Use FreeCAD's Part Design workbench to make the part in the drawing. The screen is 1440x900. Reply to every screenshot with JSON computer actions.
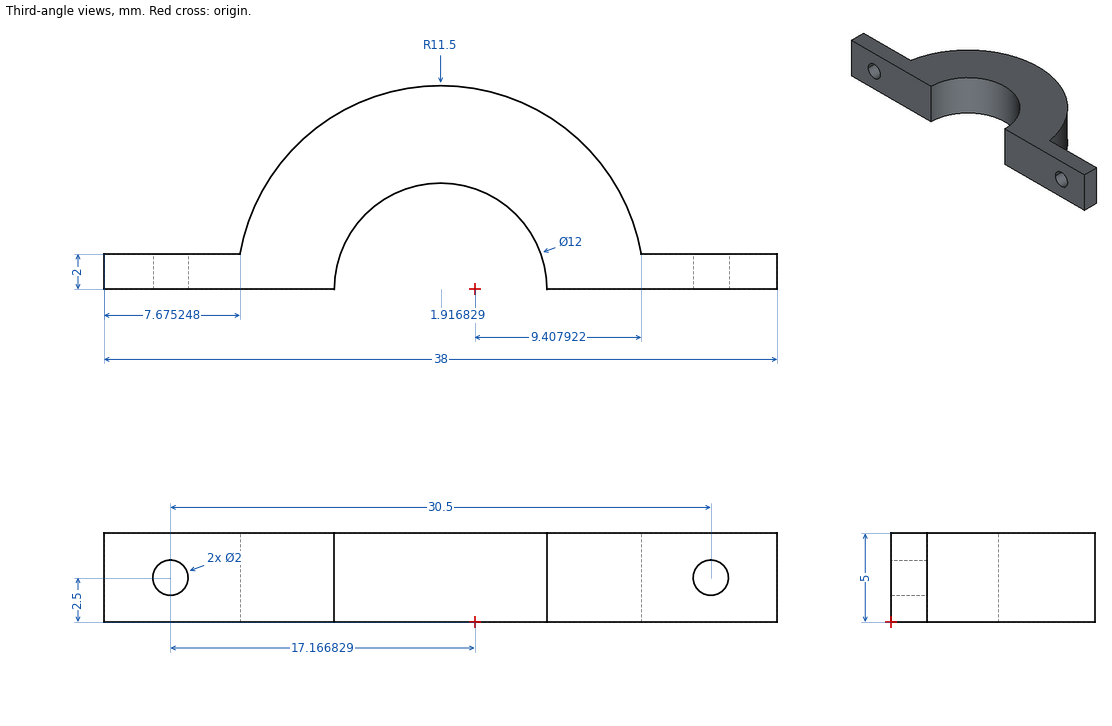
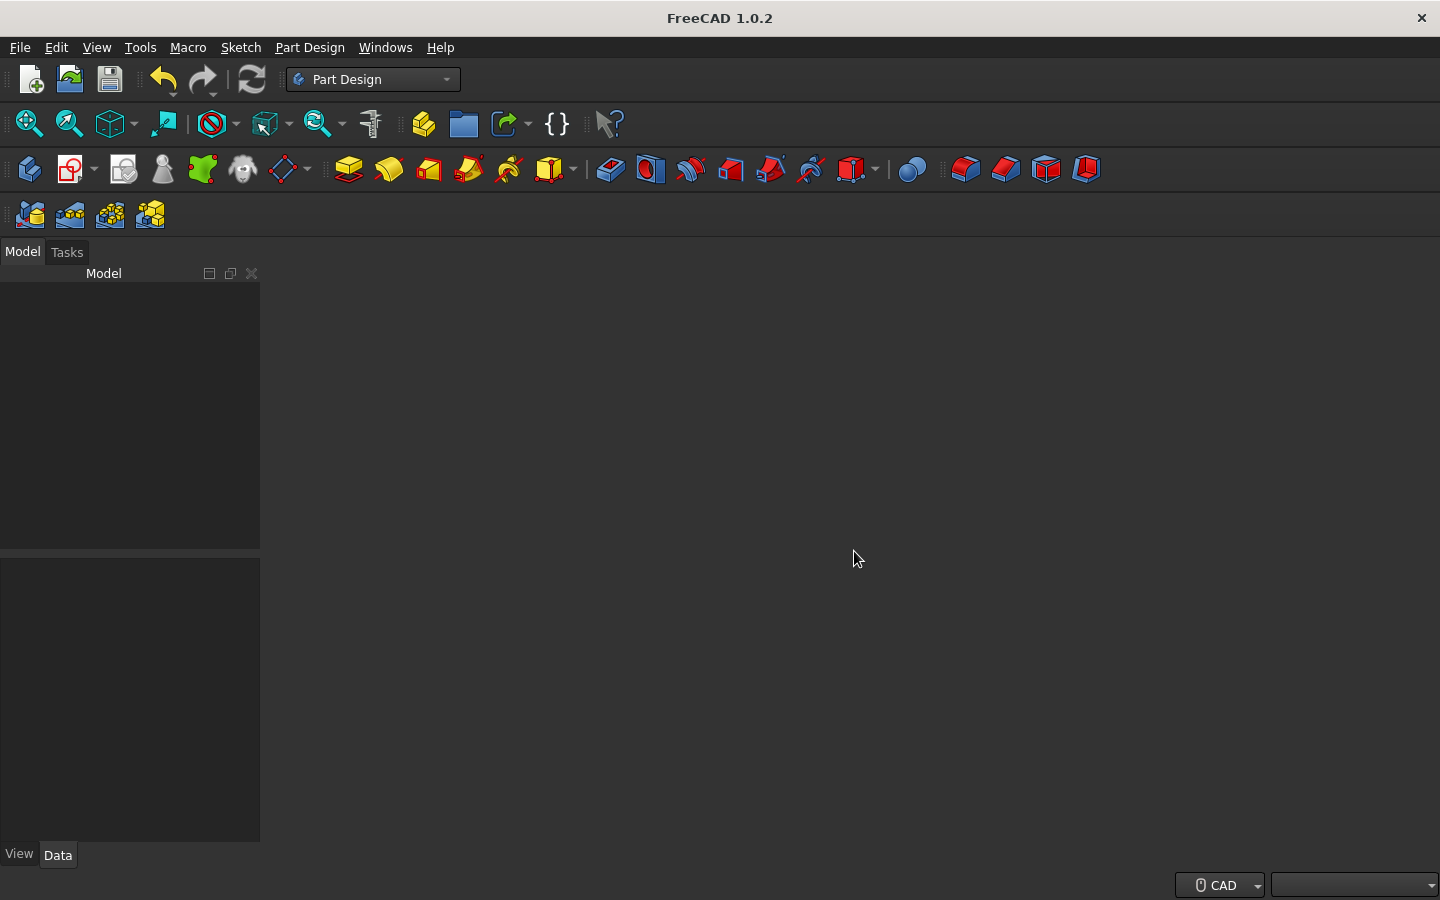
{"action": "left_click", "coordinate": [30, 80]}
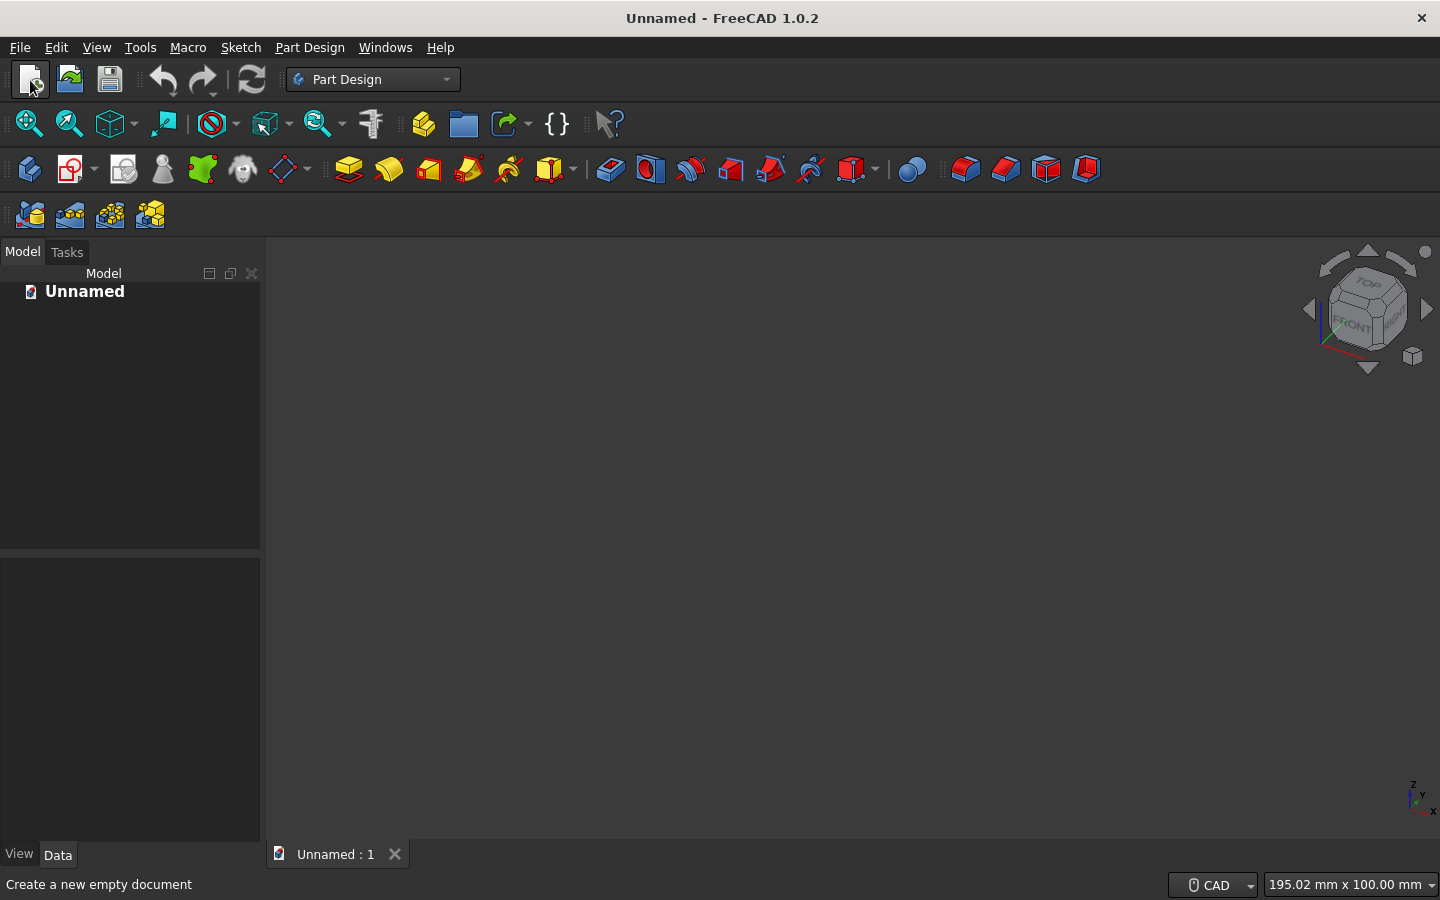
{"action": "left_click", "coordinate": [70, 170]}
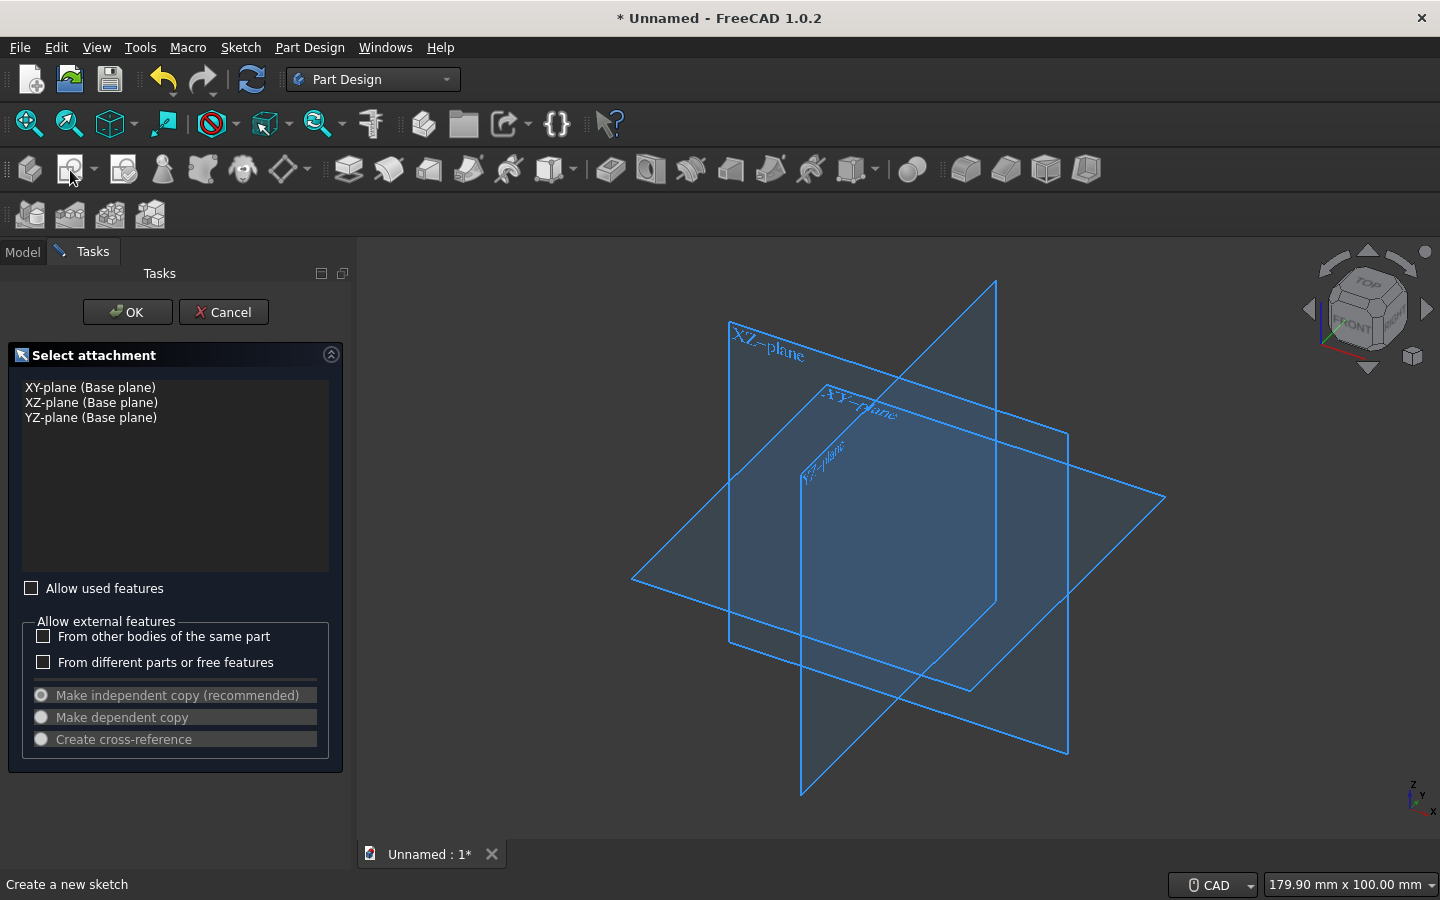
{"action": "left_click", "coordinate": [82, 388]}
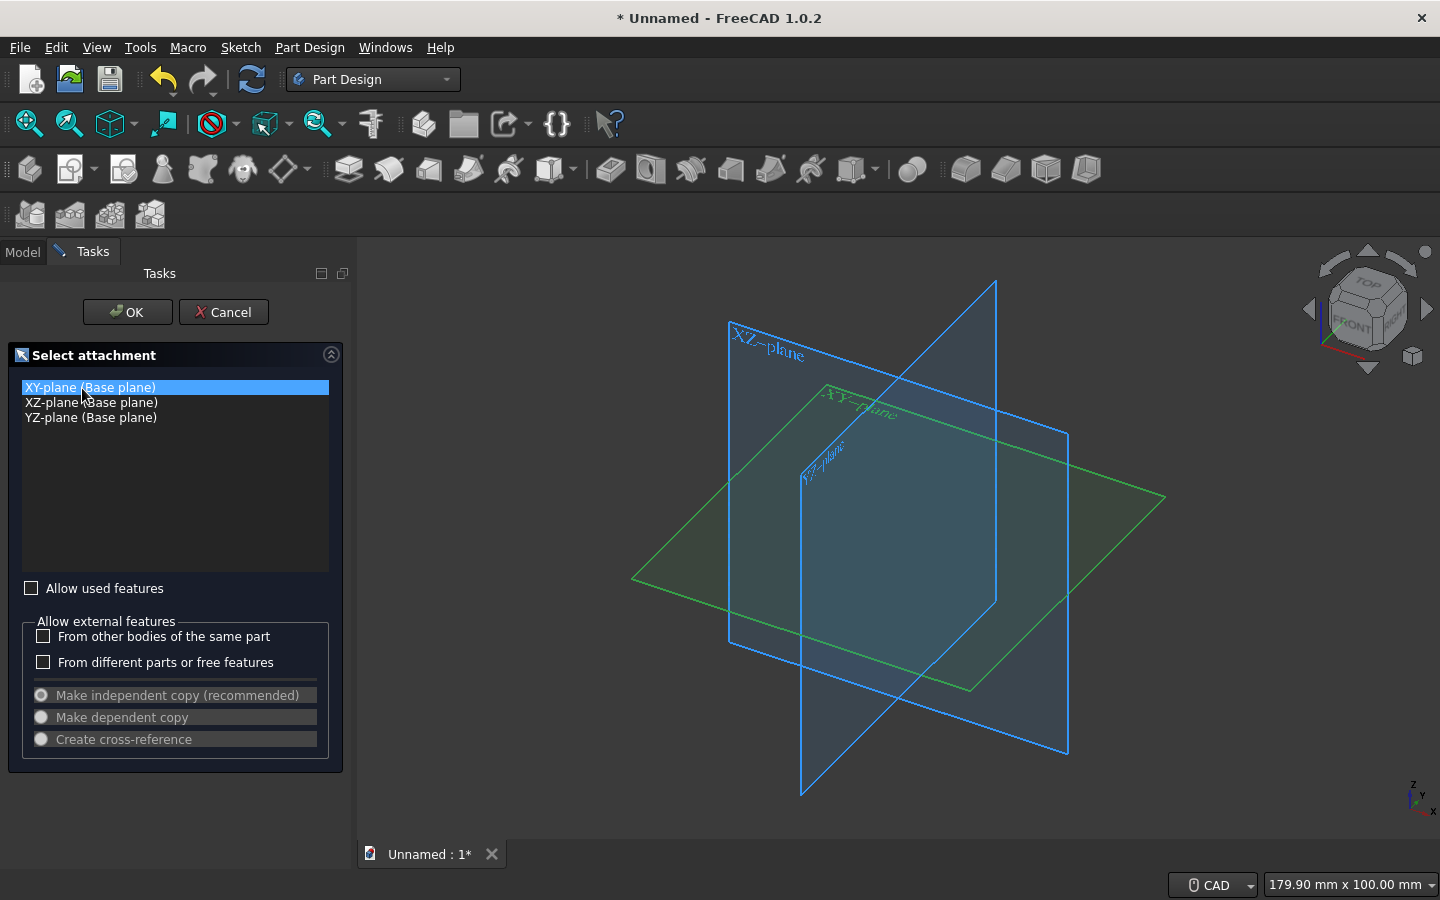
{"action": "left_click", "coordinate": [128, 312]}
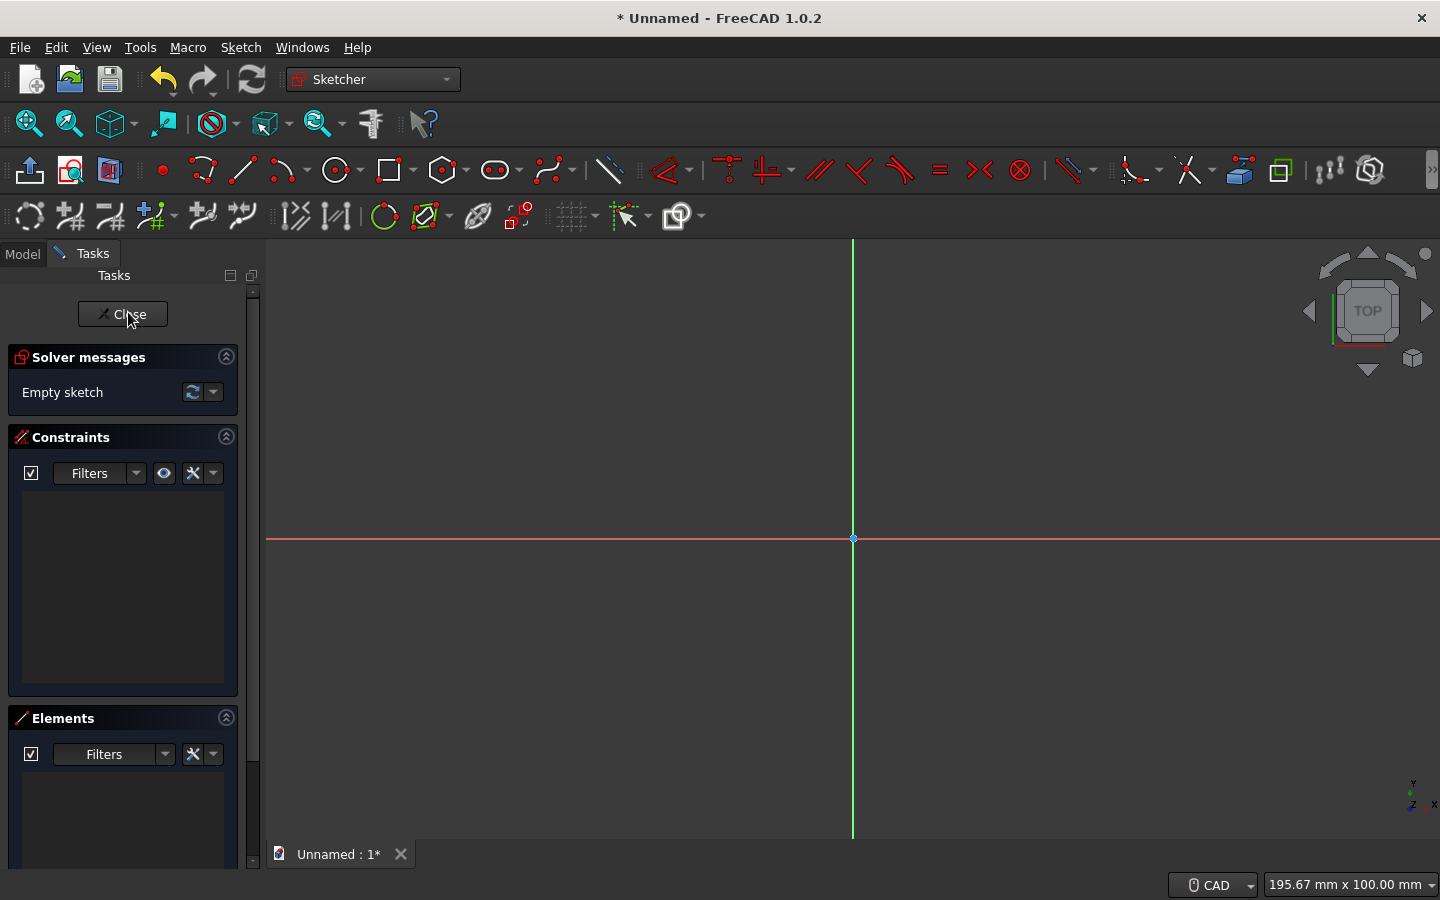
{"action": "scroll", "coordinate": [866, 490], "scroll_direction": "up", "scroll_amount": 6}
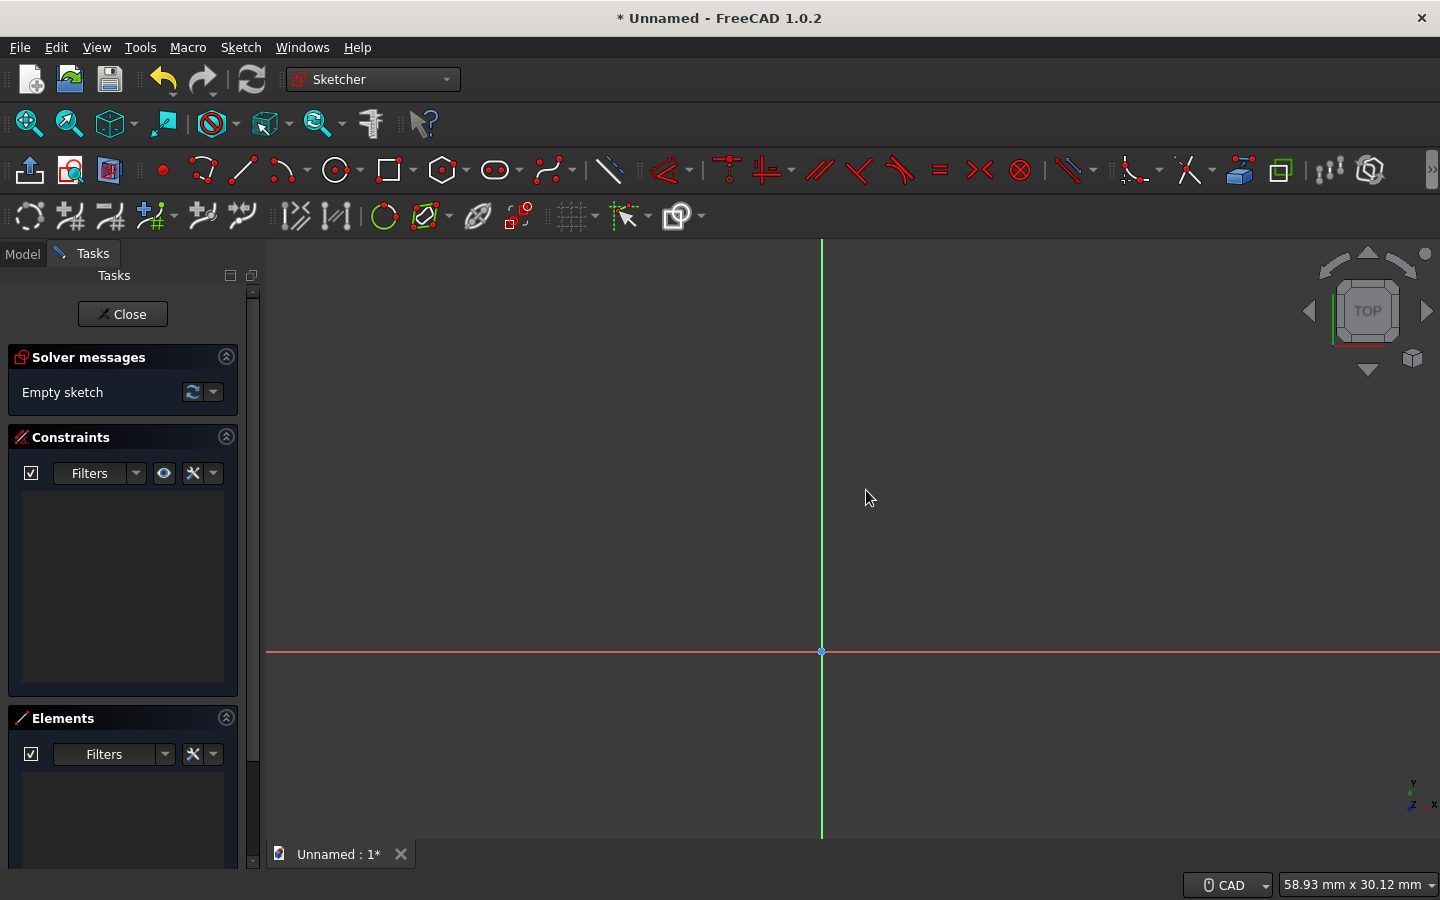
{"action": "key", "text": "g m"}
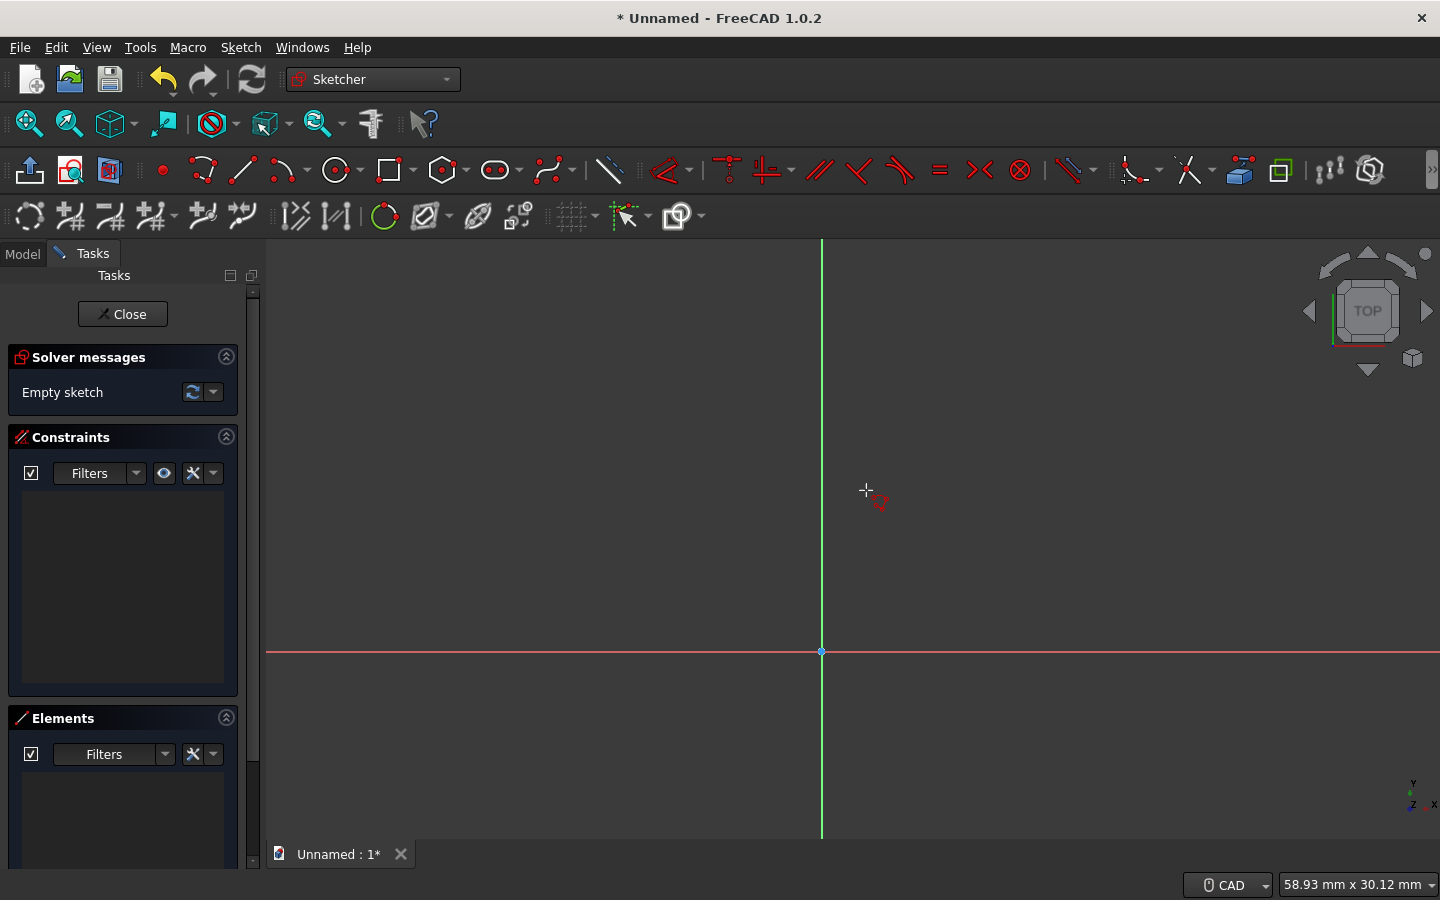
{"action": "left_click", "coordinate": [558, 612]}
{"action": "left_click", "coordinate": [405, 612]}
{"action": "left_click", "coordinate": [405, 652]}
{"action": "left_click", "coordinate": [1162, 643]}
{"action": "left_click", "coordinate": [1162, 612]}
{"action": "left_click", "coordinate": [1009, 612]}
{"action": "right_click", "coordinate": [1009, 612]}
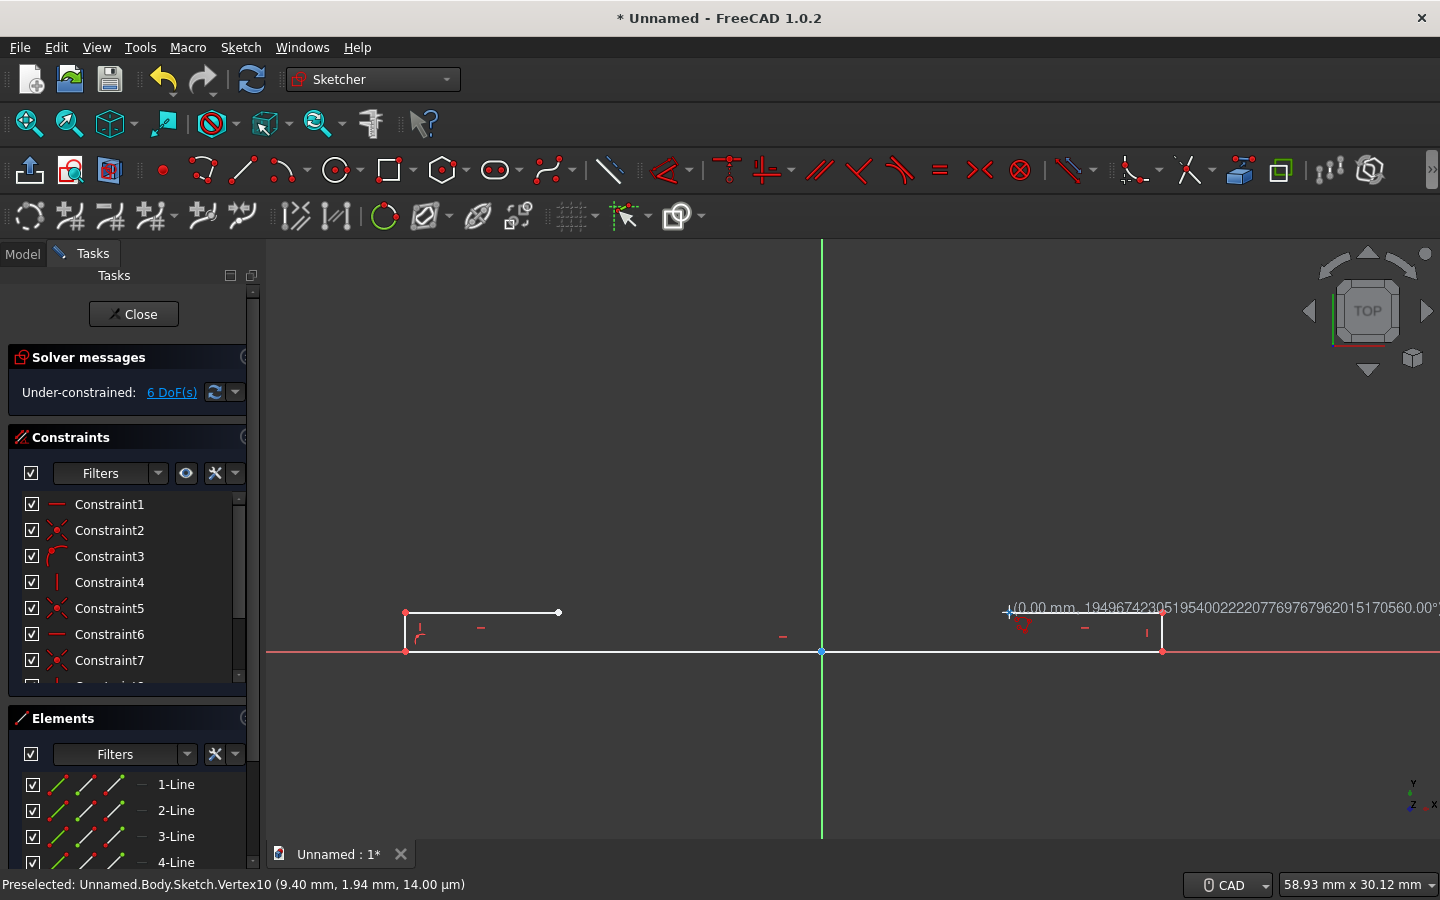
{"action": "key", "text": "g 3 a"}